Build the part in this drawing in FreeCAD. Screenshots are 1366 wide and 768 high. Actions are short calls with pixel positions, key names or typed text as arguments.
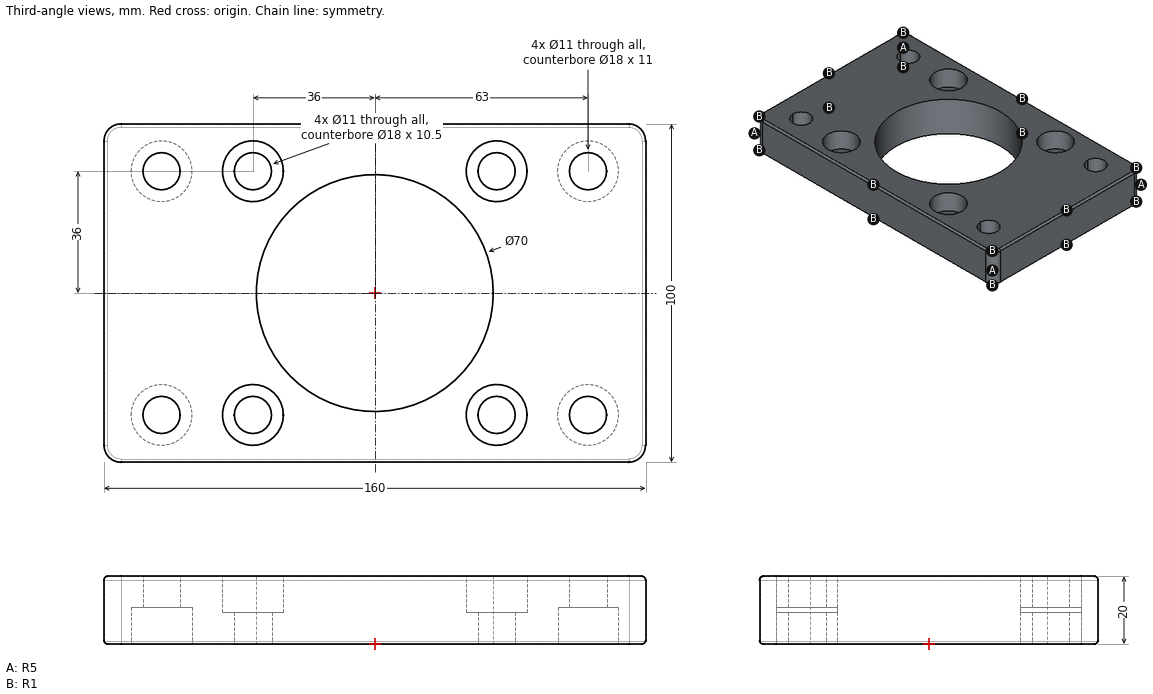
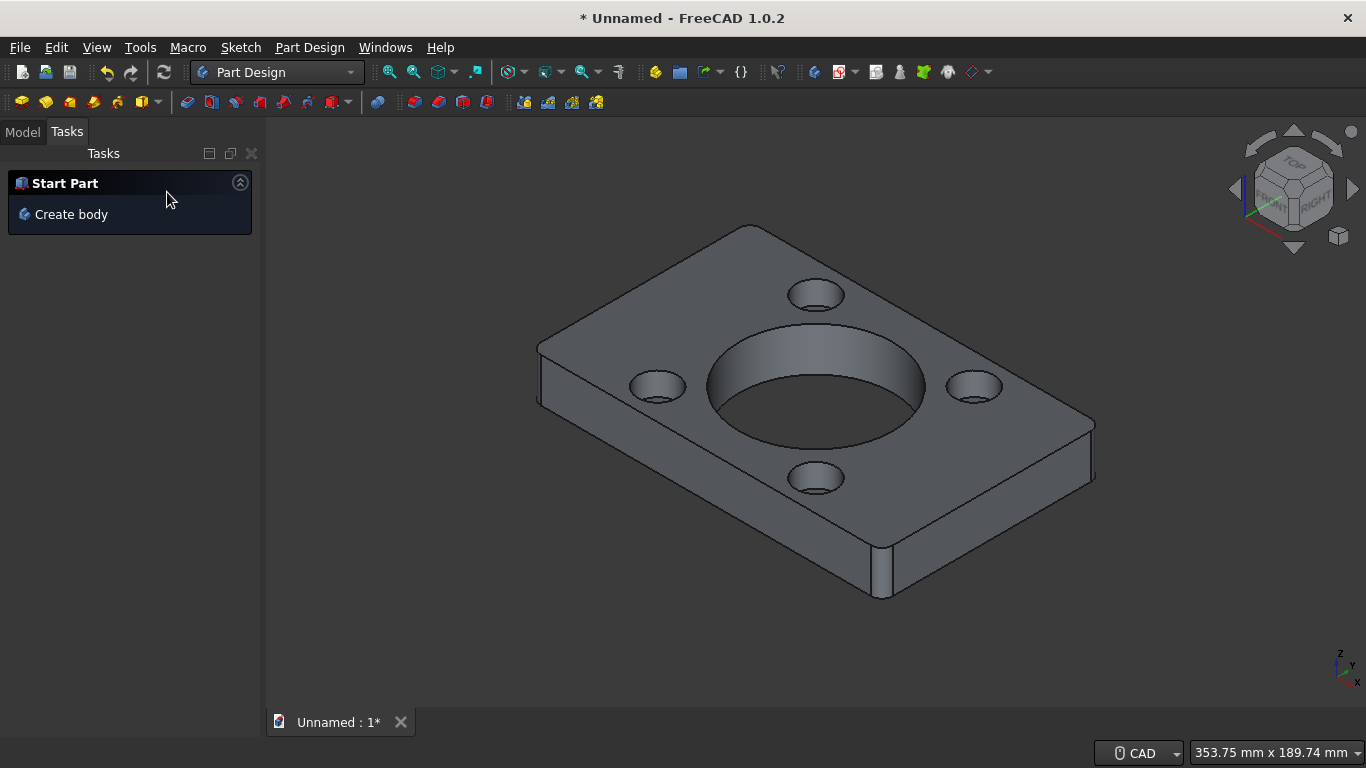
click(840, 72)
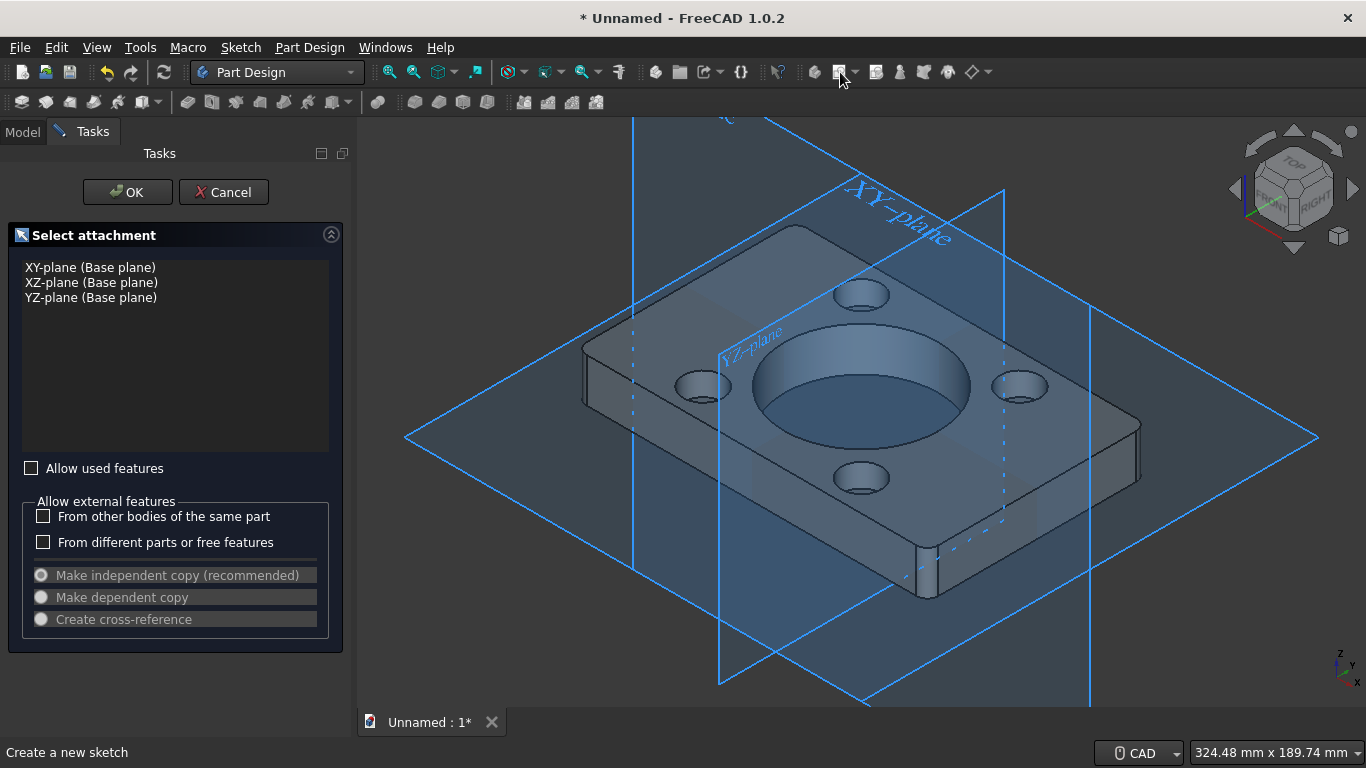
click(82, 268)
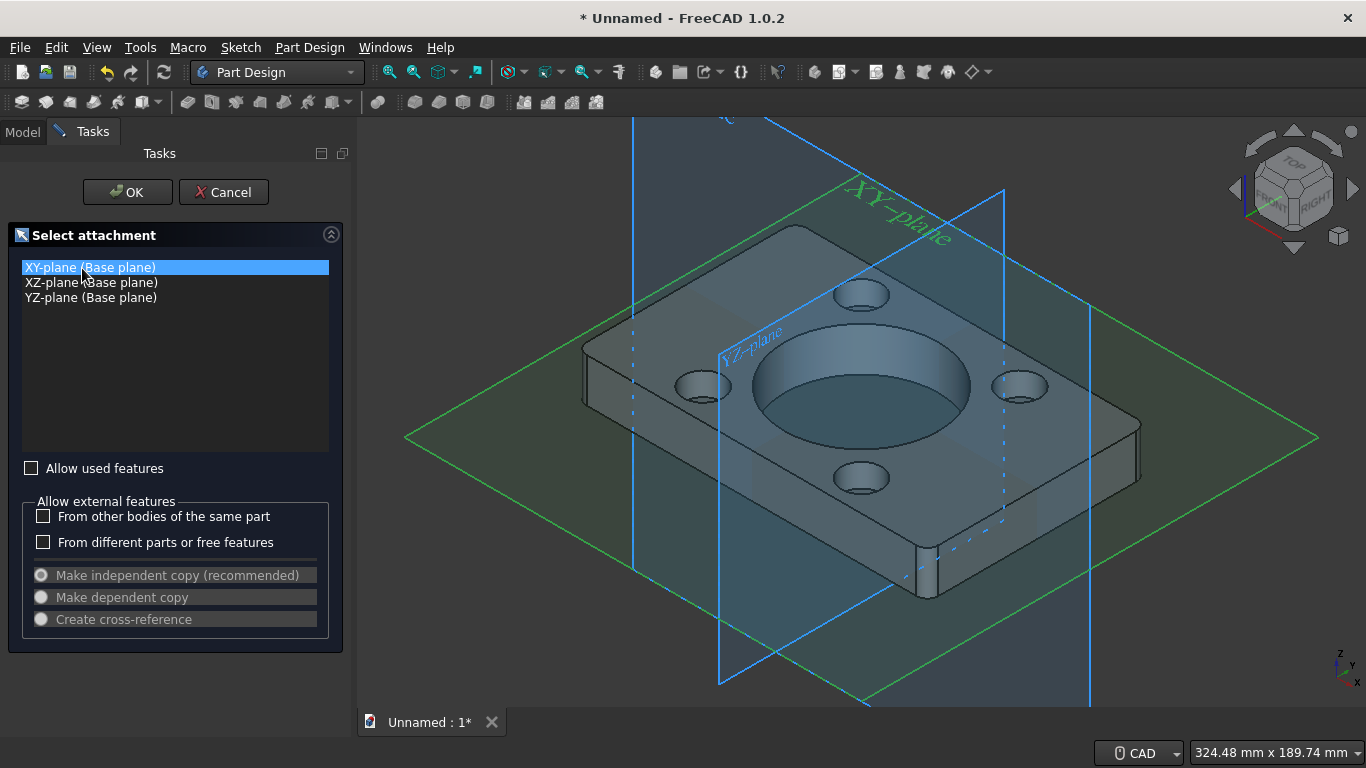
click(128, 192)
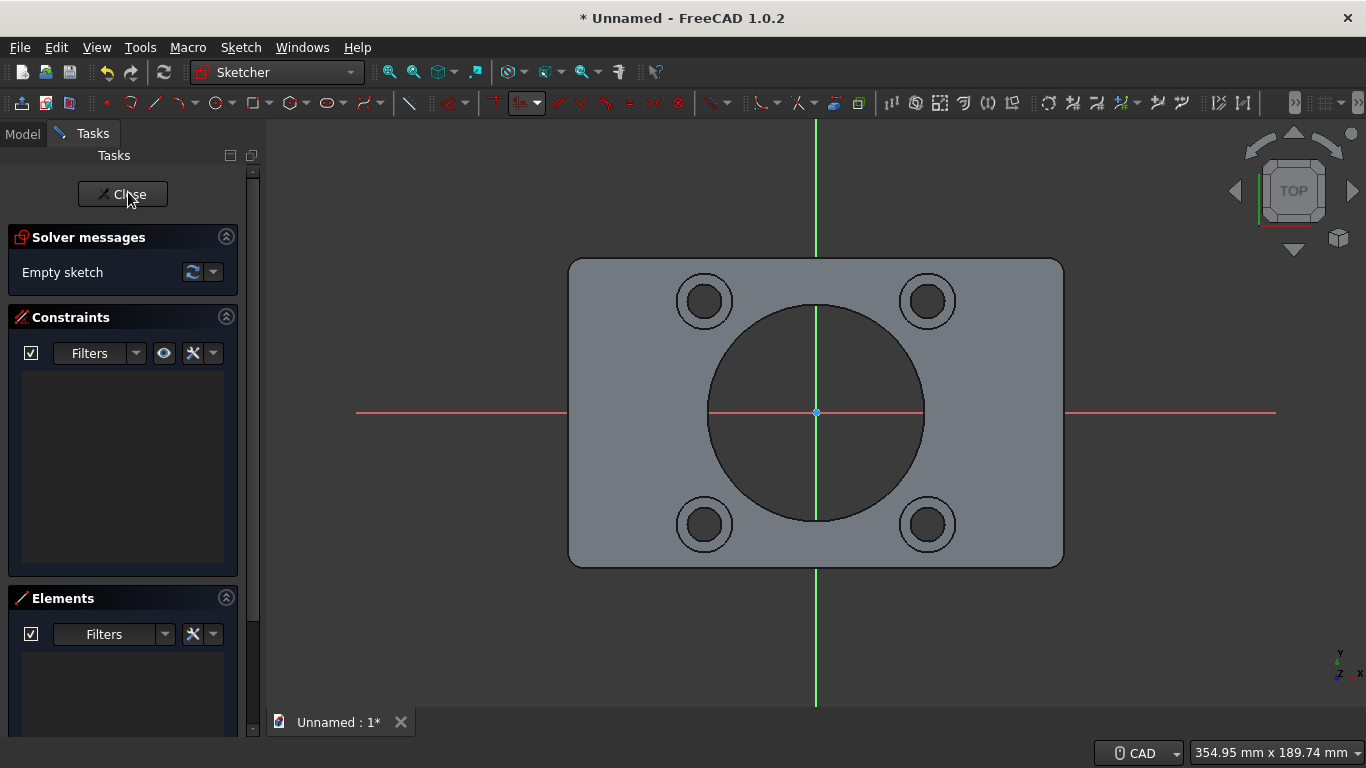
click(70, 104)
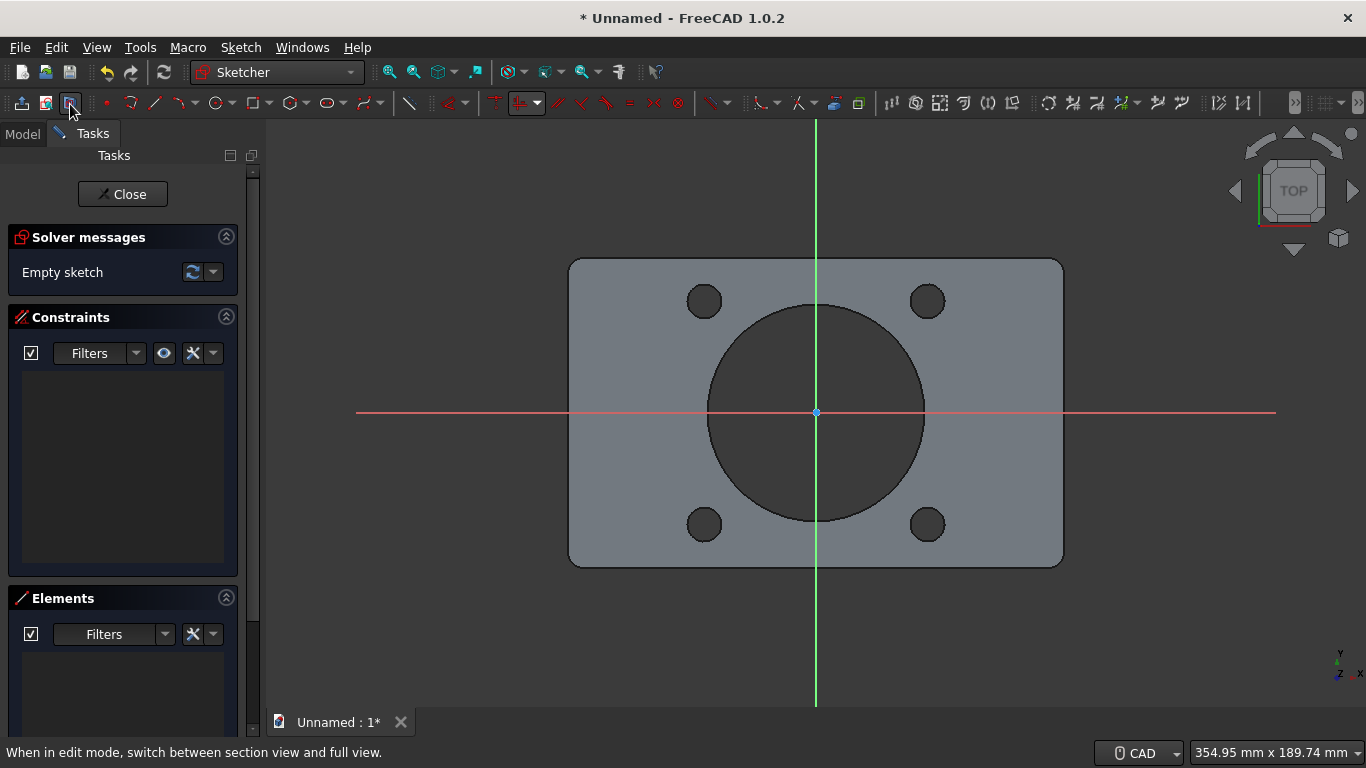
scroll(955, 413, up, 2)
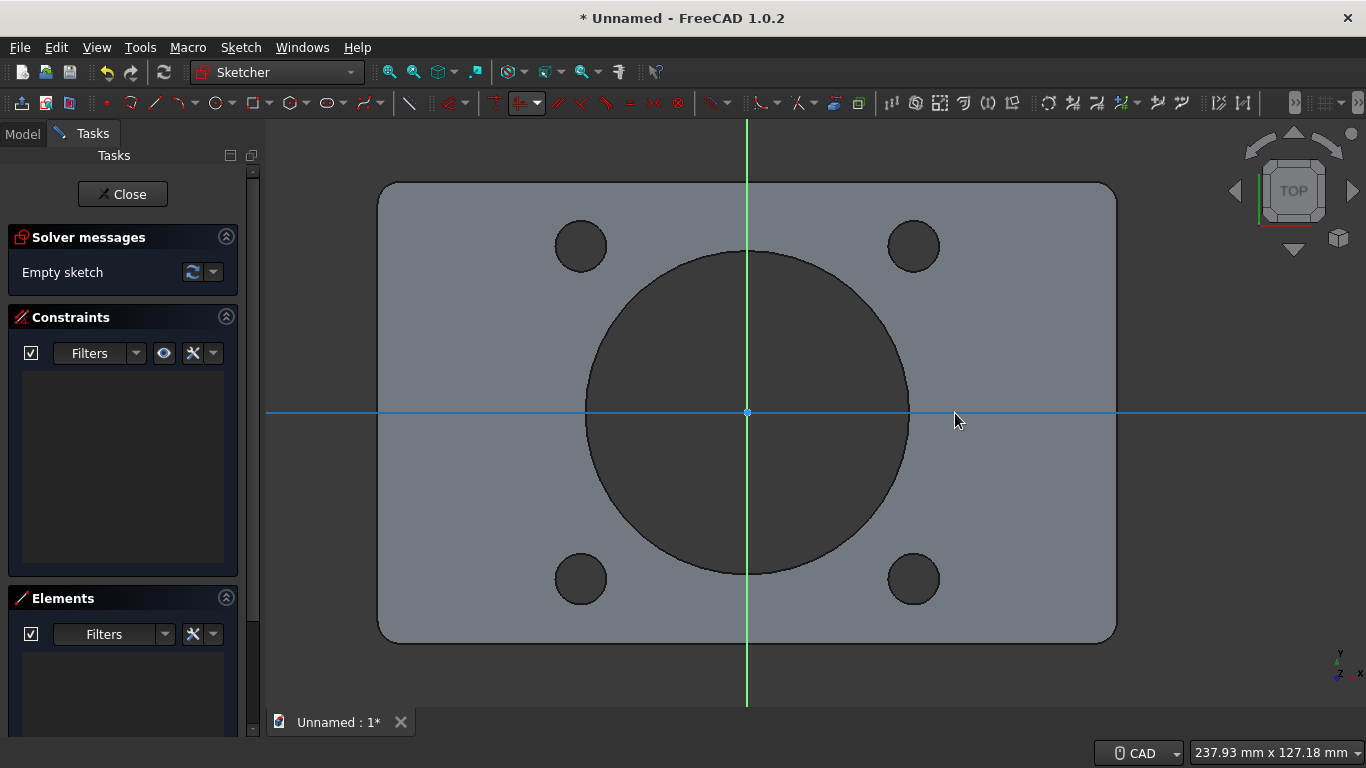
key(g)
key(c)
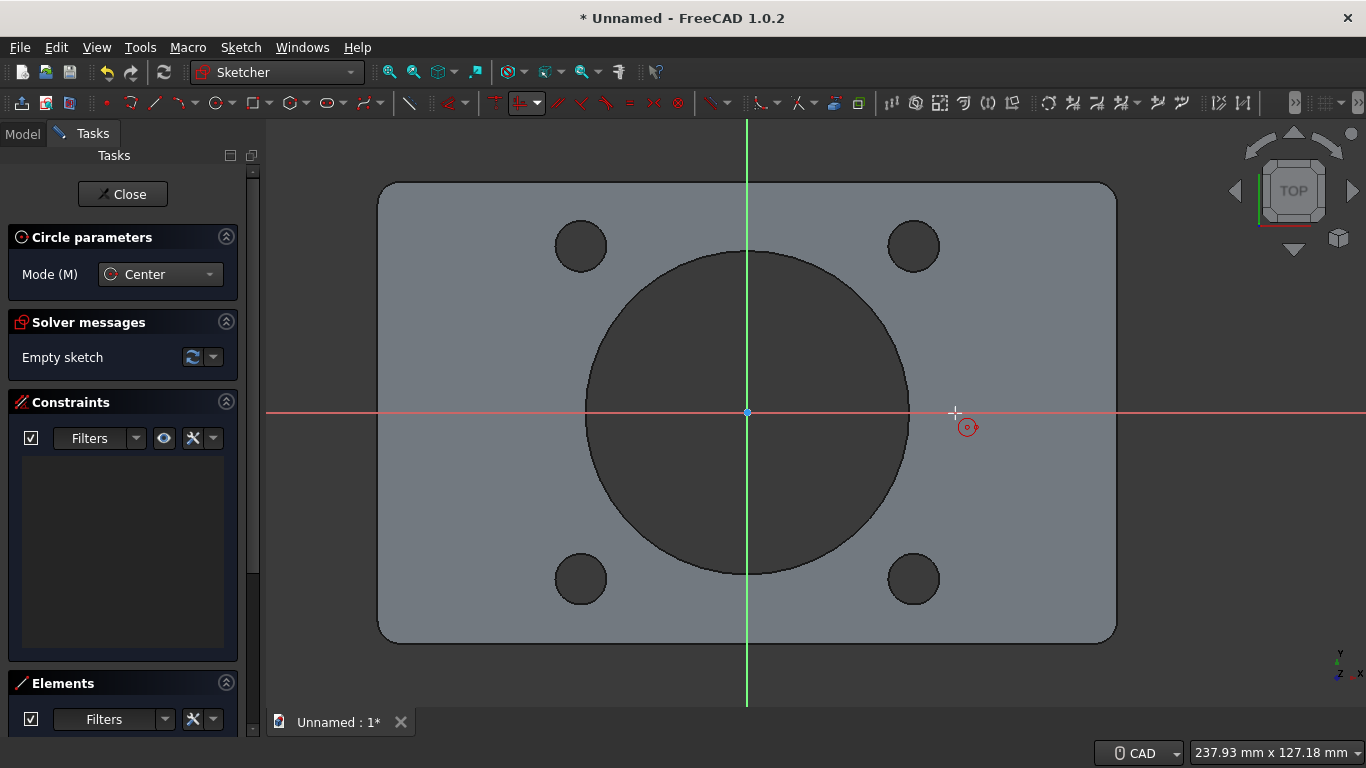
click(1039, 246)
click(1057, 228)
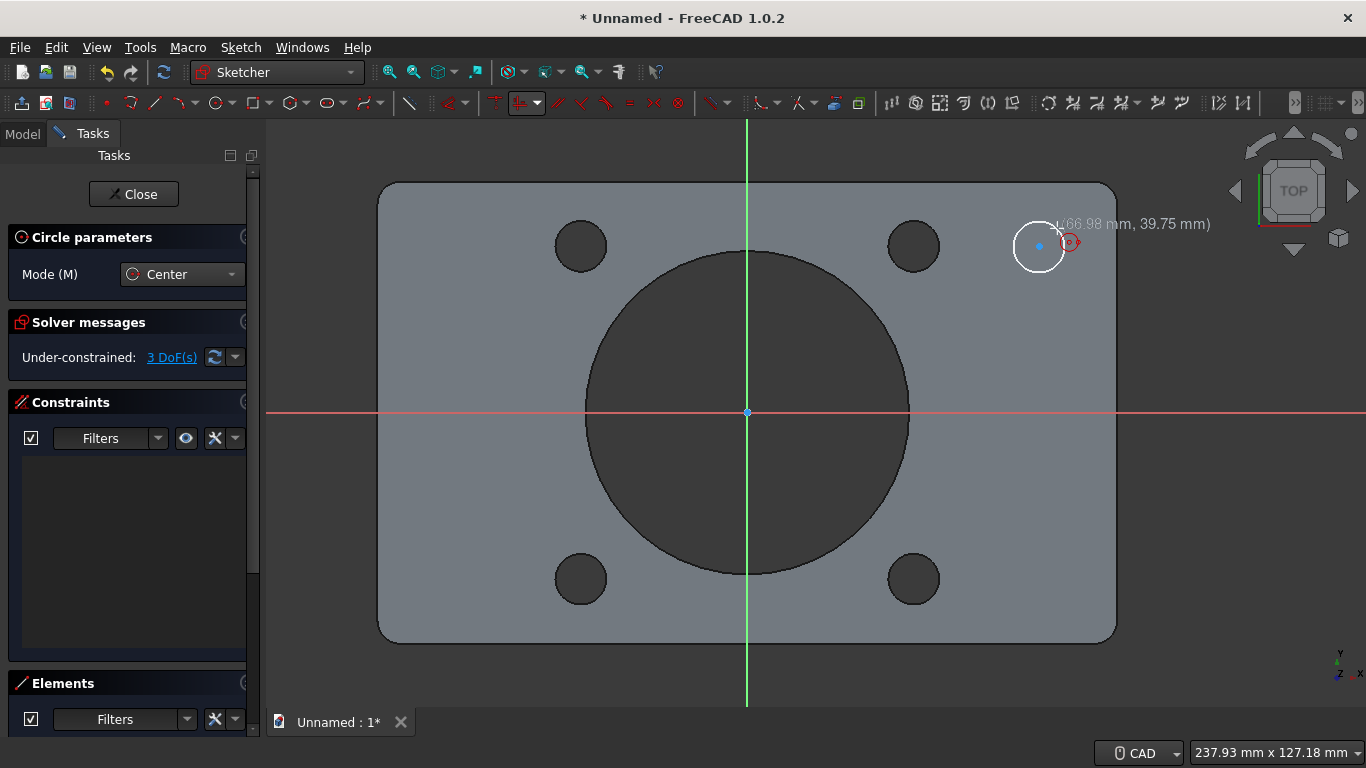
click(456, 246)
click(474, 228)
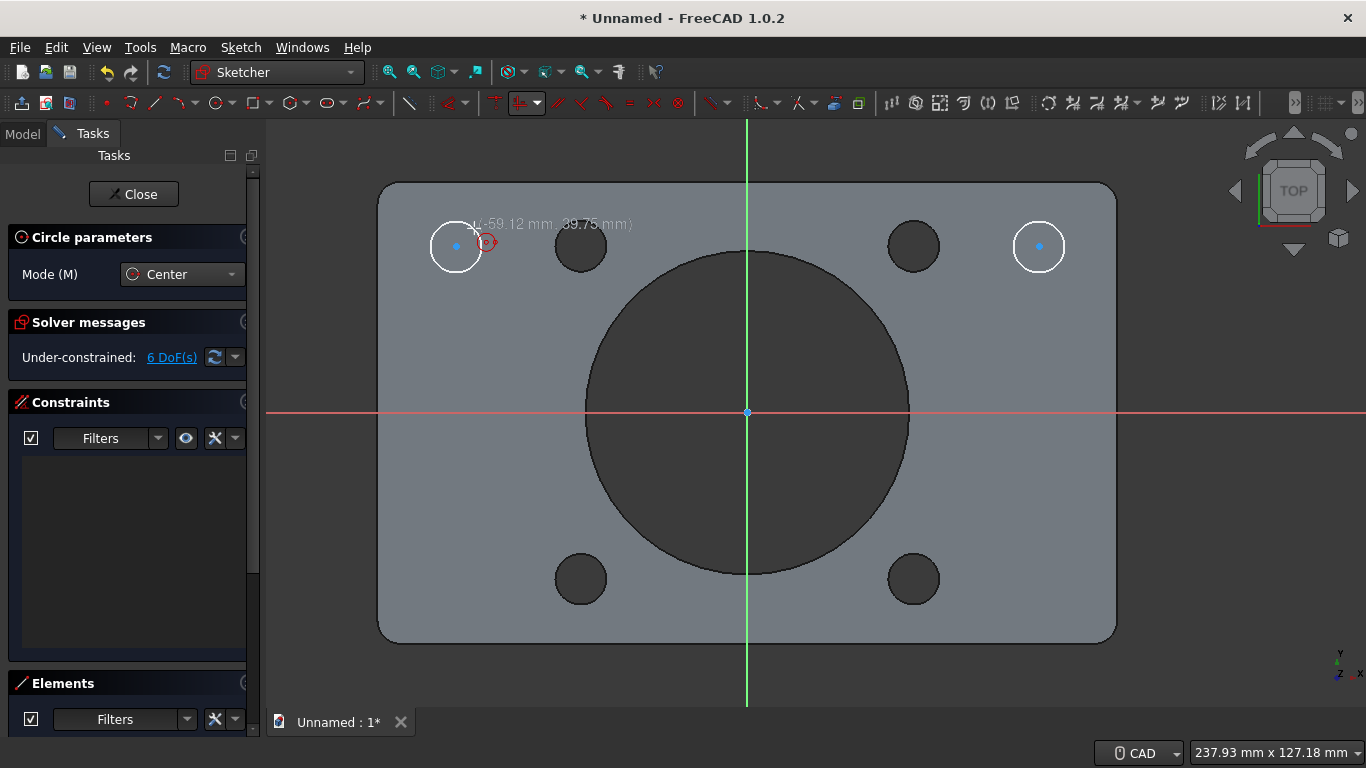
click(1039, 579)
click(1057, 561)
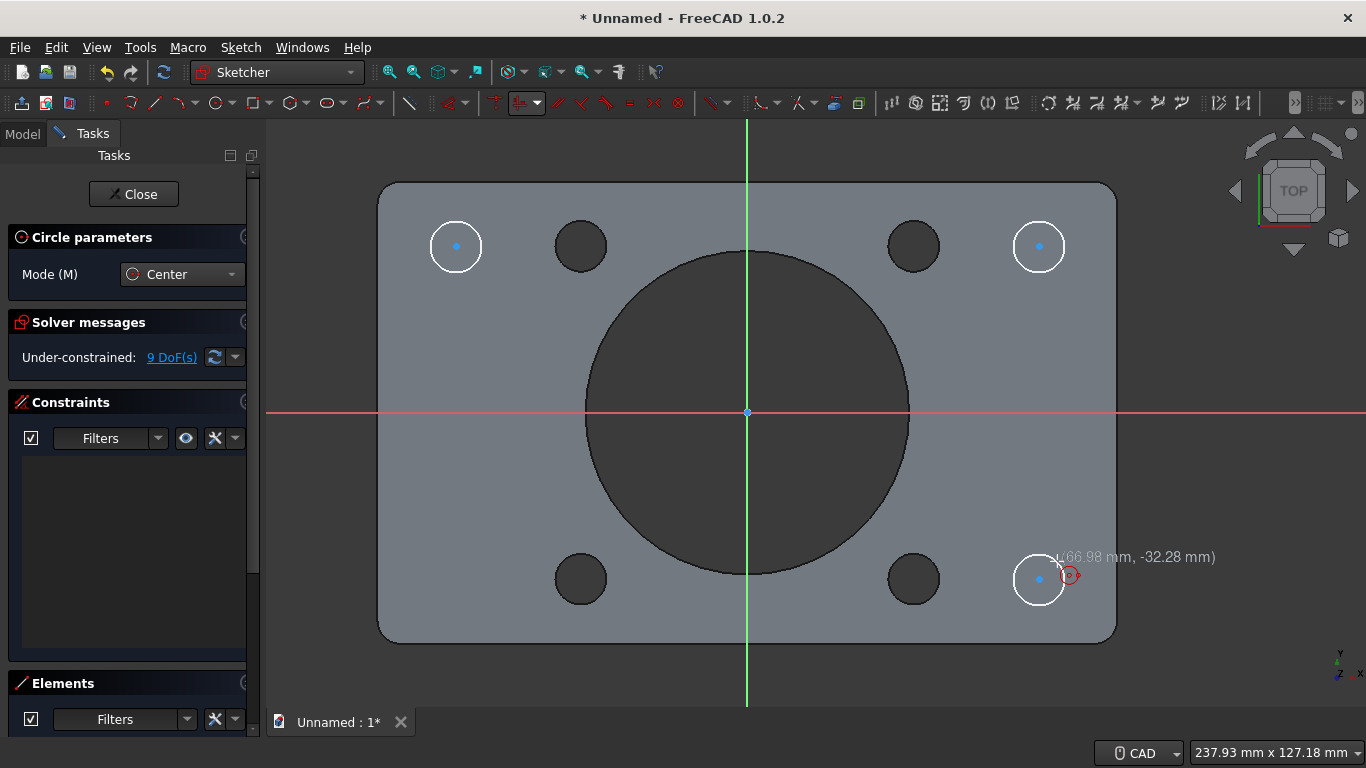
click(456, 579)
click(474, 561)
key(Escape)